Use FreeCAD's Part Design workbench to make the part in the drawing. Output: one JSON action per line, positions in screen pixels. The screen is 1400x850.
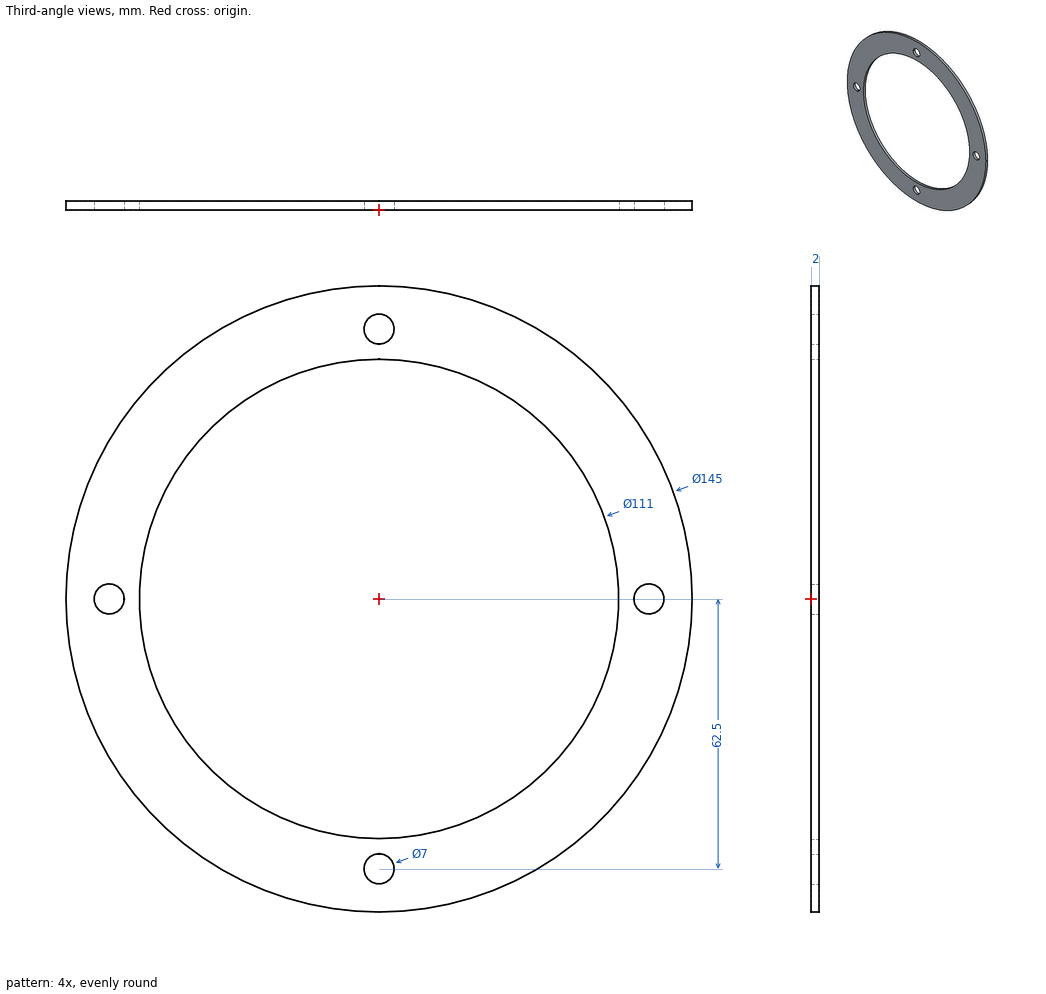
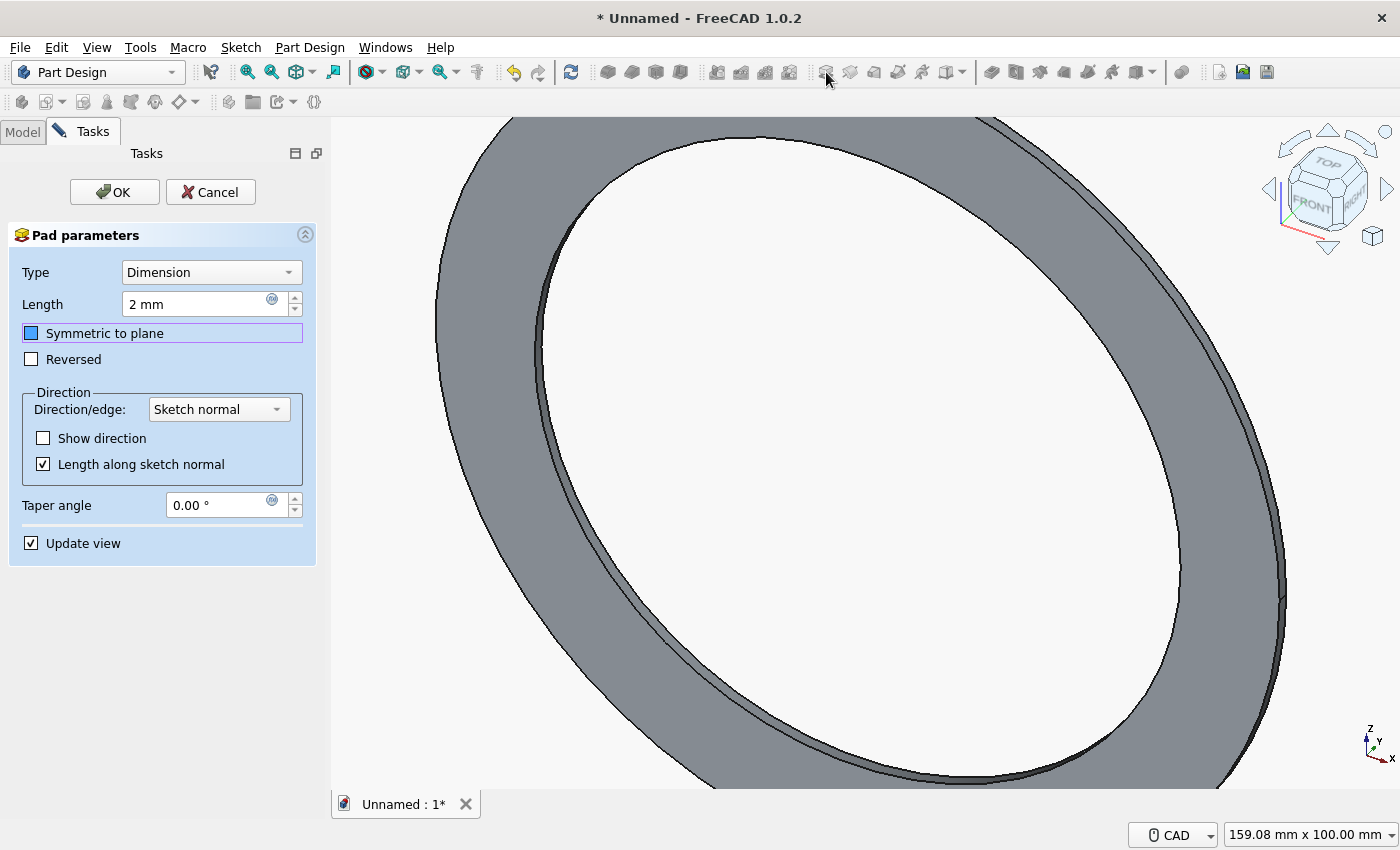
{"action": "left_click", "coordinate": [30, 359]}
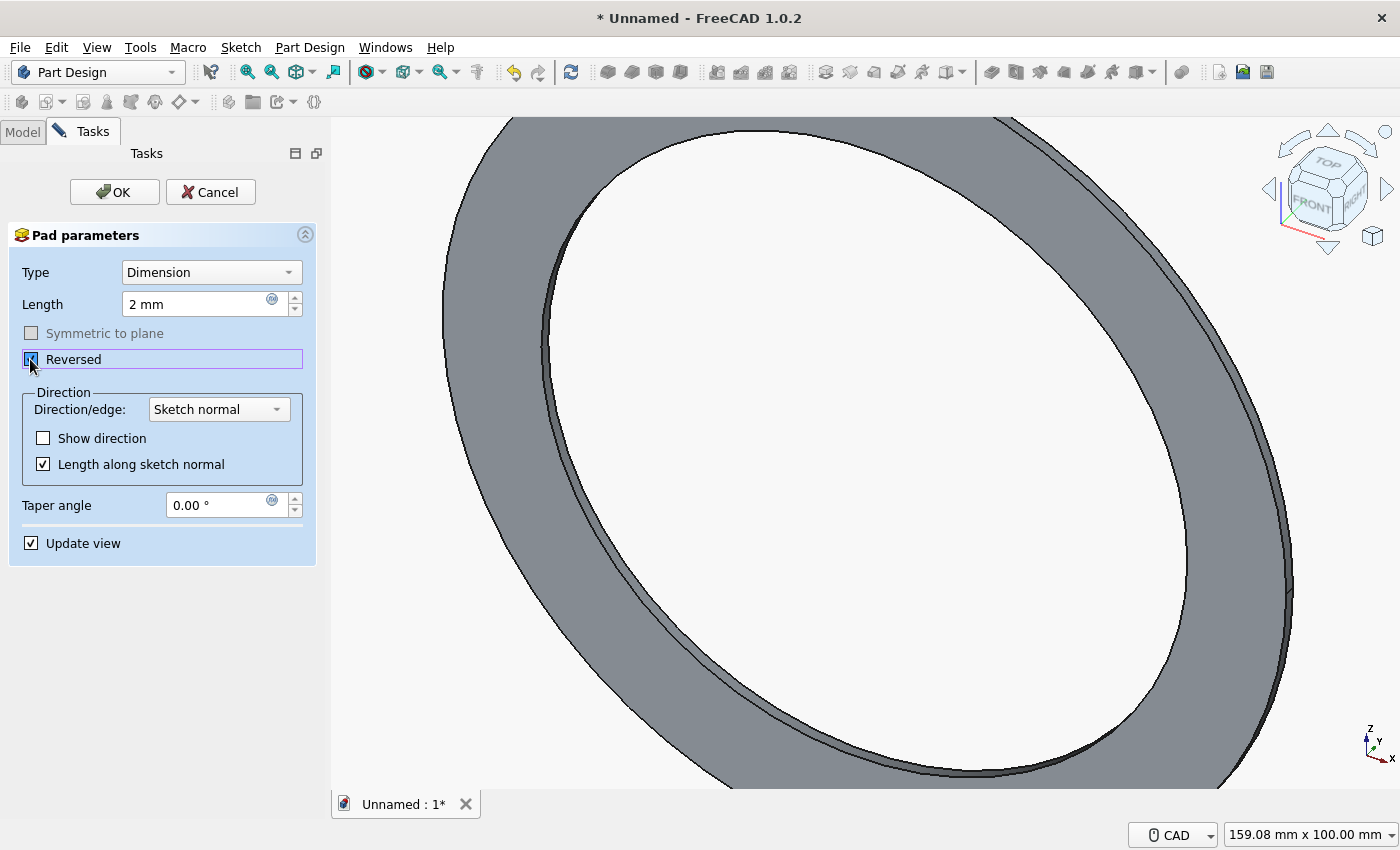
{"action": "left_click", "coordinate": [115, 192]}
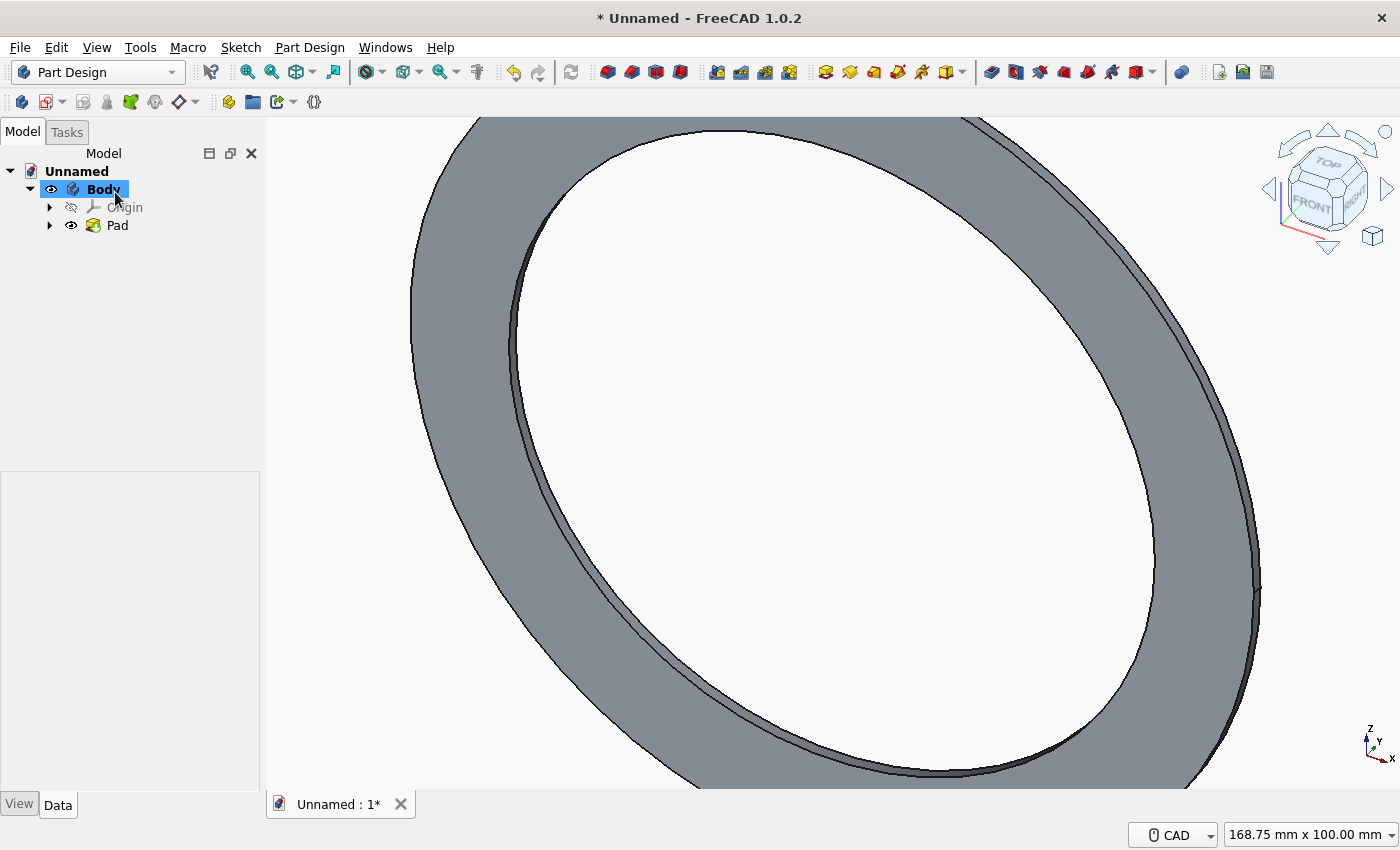
{"action": "left_click", "coordinate": [248, 72]}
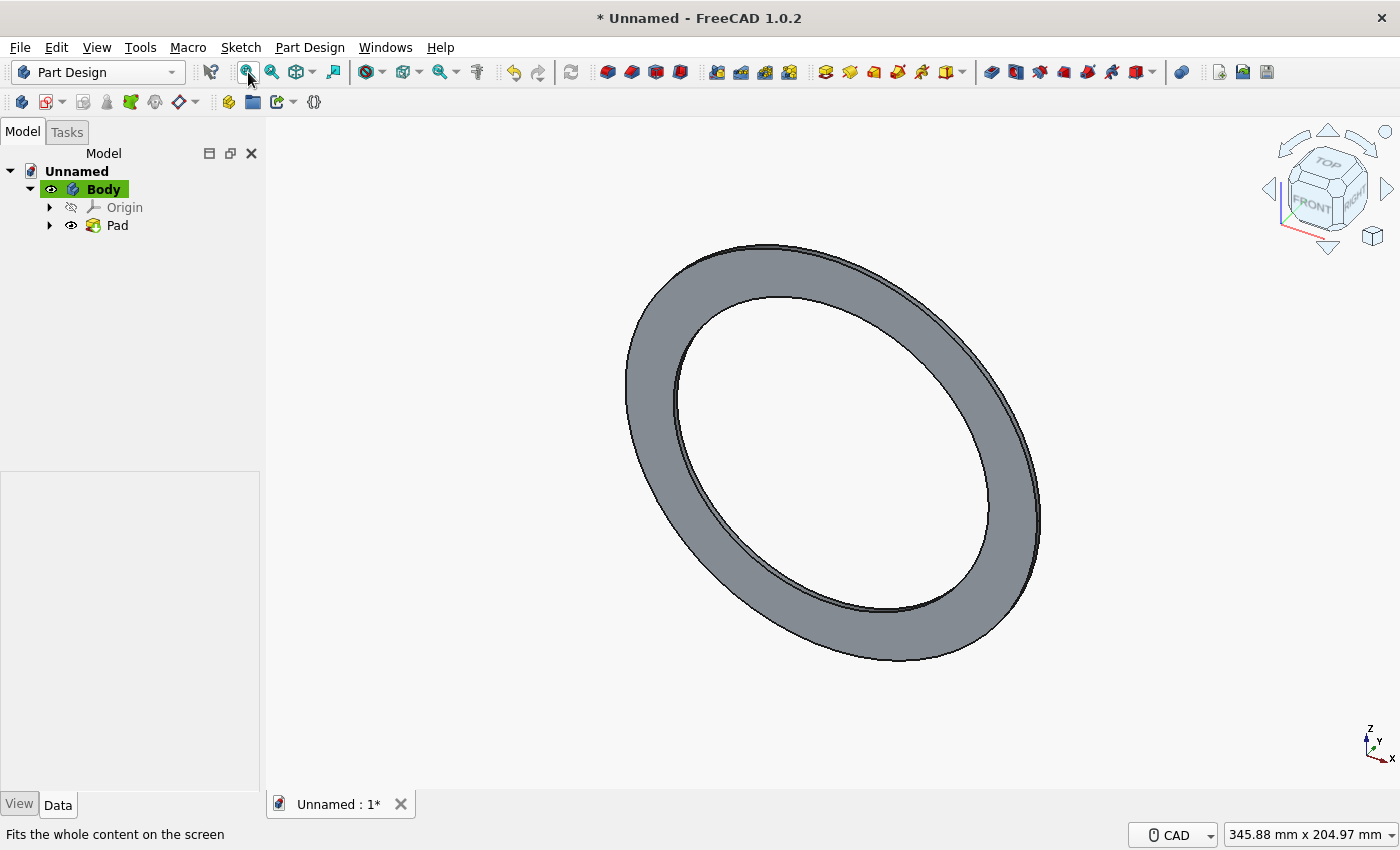
{"action": "key", "text": "4"}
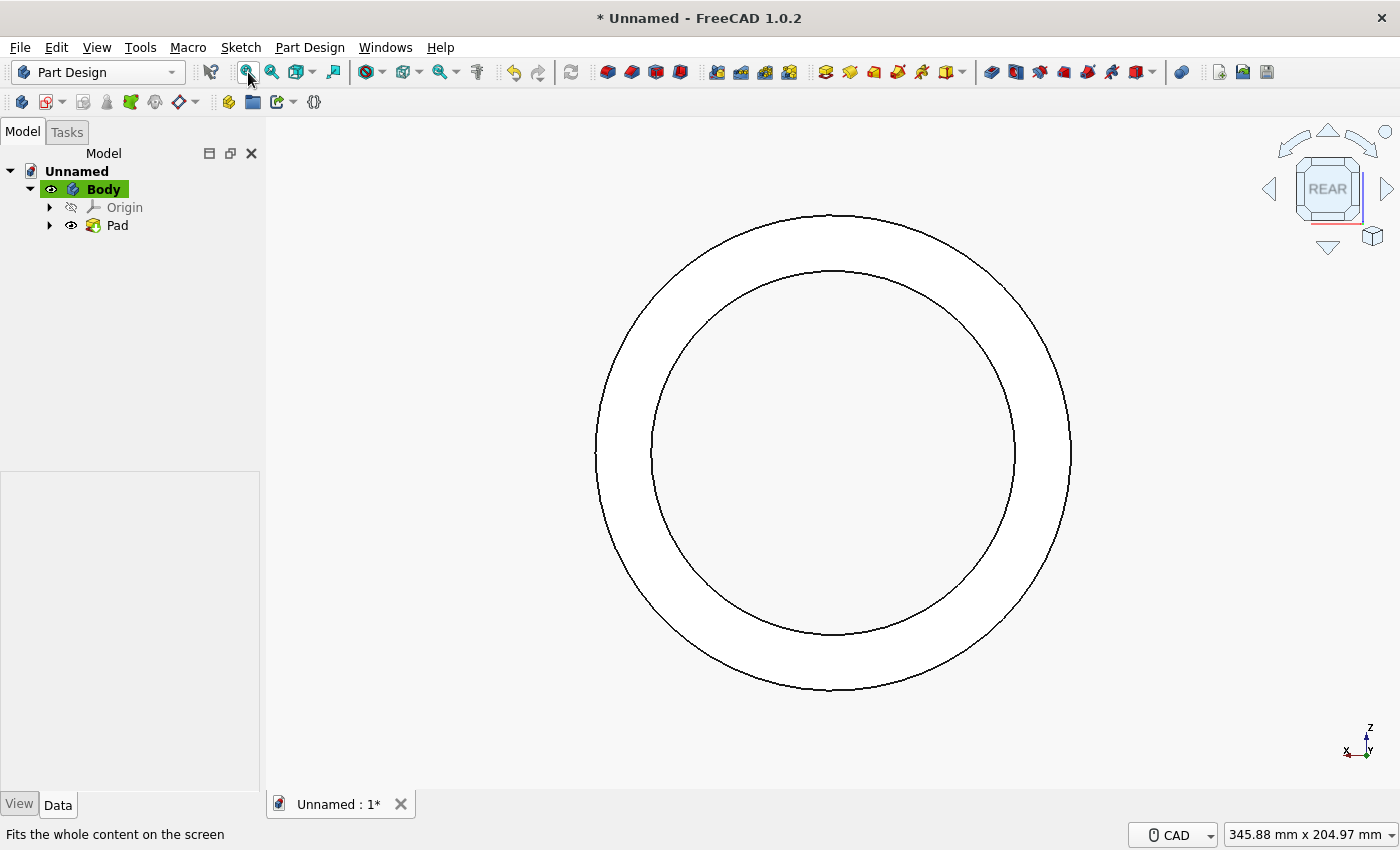
{"action": "left_click", "coordinate": [629, 520]}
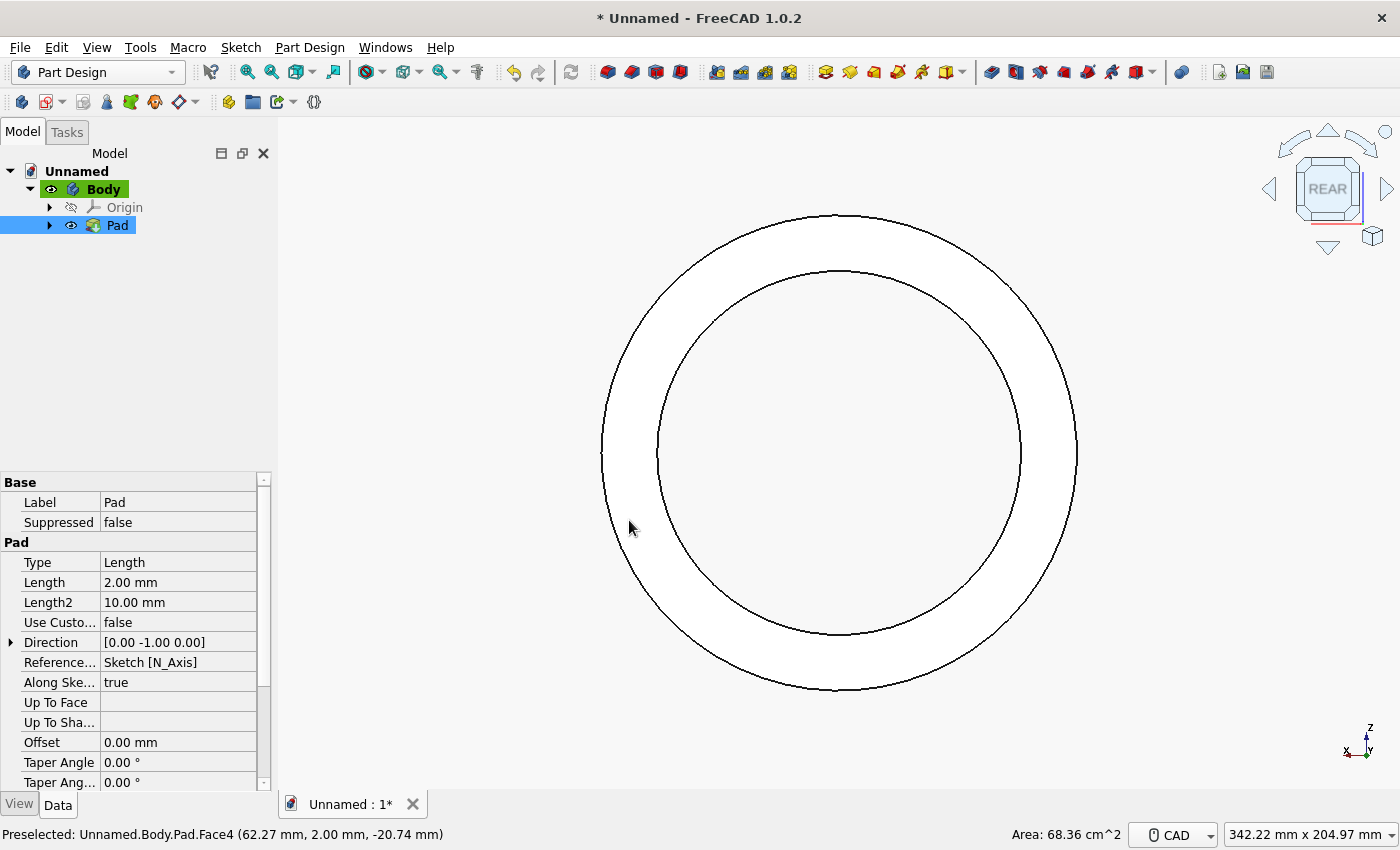
{"action": "left_click", "coordinate": [46, 102]}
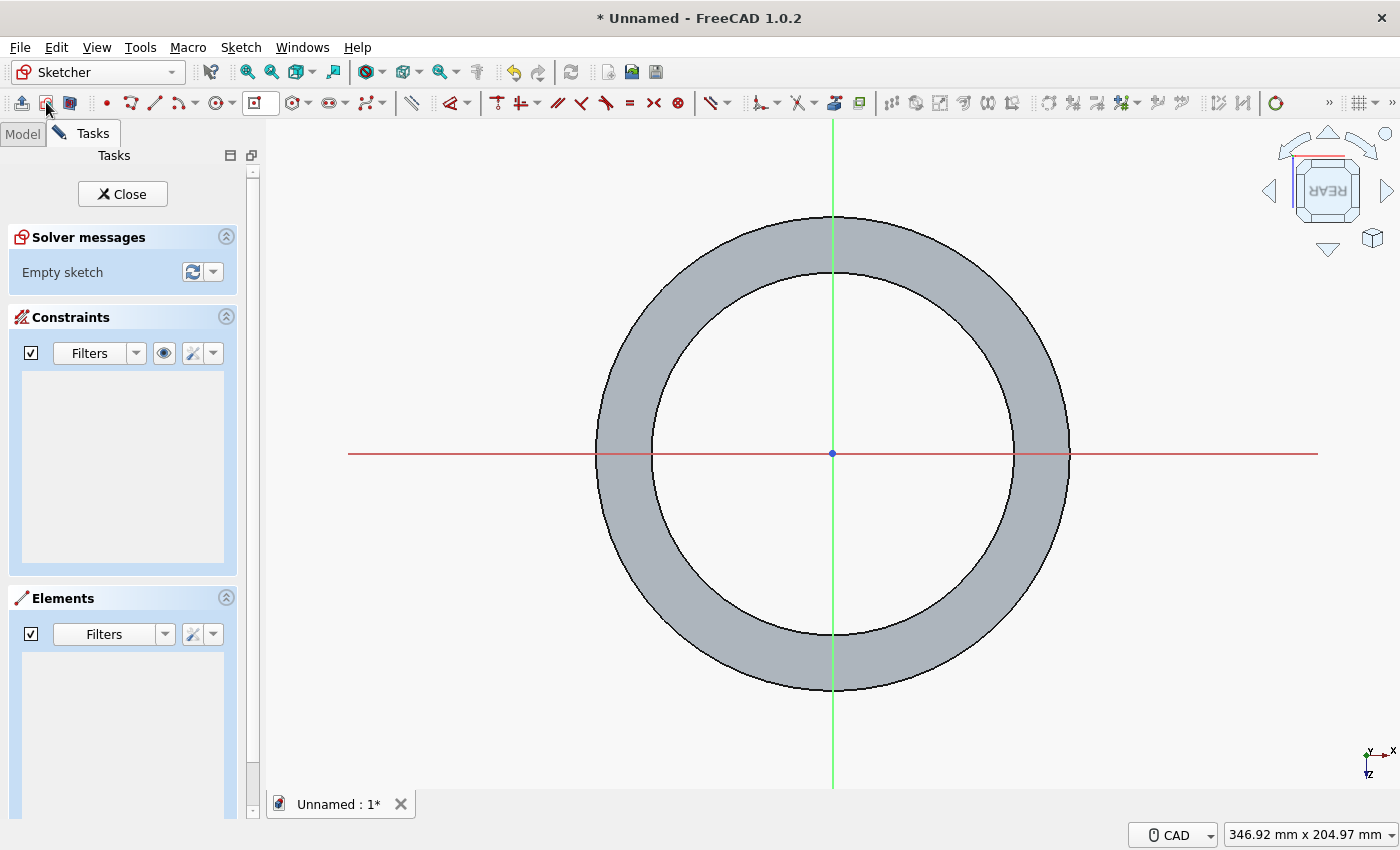
{"action": "scroll", "coordinate": [836, 239], "scroll_direction": "up", "scroll_amount": 15}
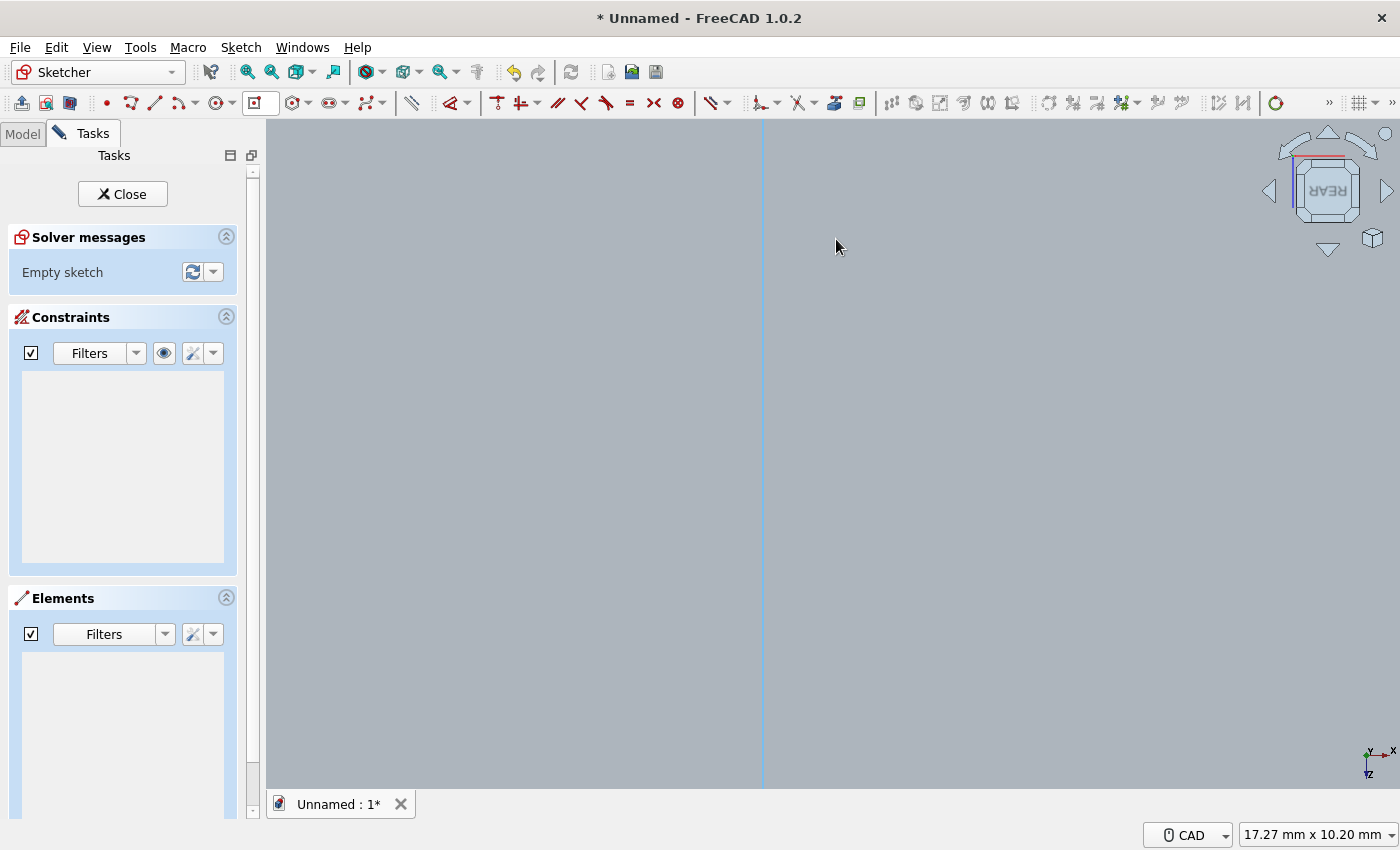
{"action": "left_click", "coordinate": [216, 104]}